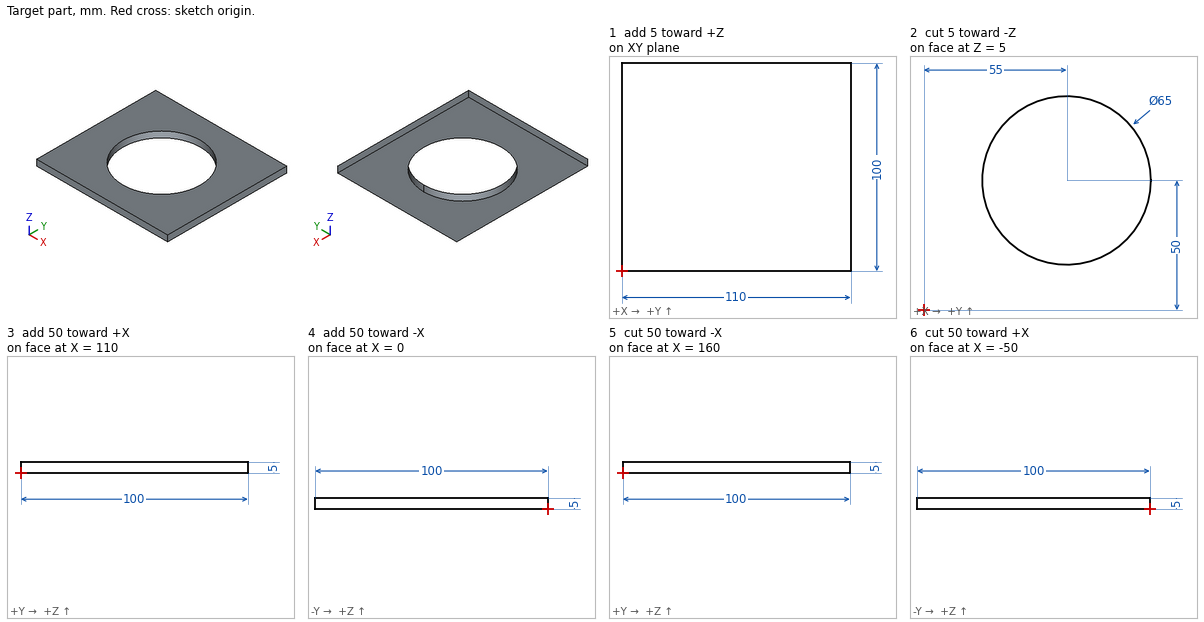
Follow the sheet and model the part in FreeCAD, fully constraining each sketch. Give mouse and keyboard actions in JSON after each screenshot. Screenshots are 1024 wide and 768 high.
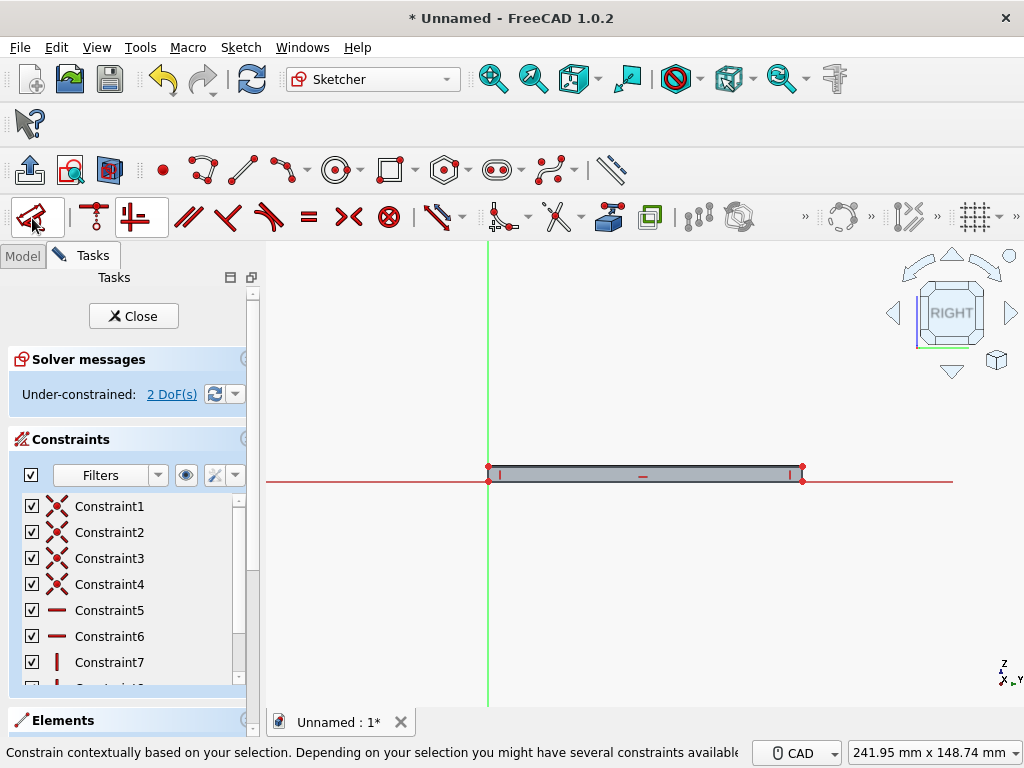
{"action": "scroll", "coordinate": [802, 474], "scroll_direction": "up", "scroll_amount": 5}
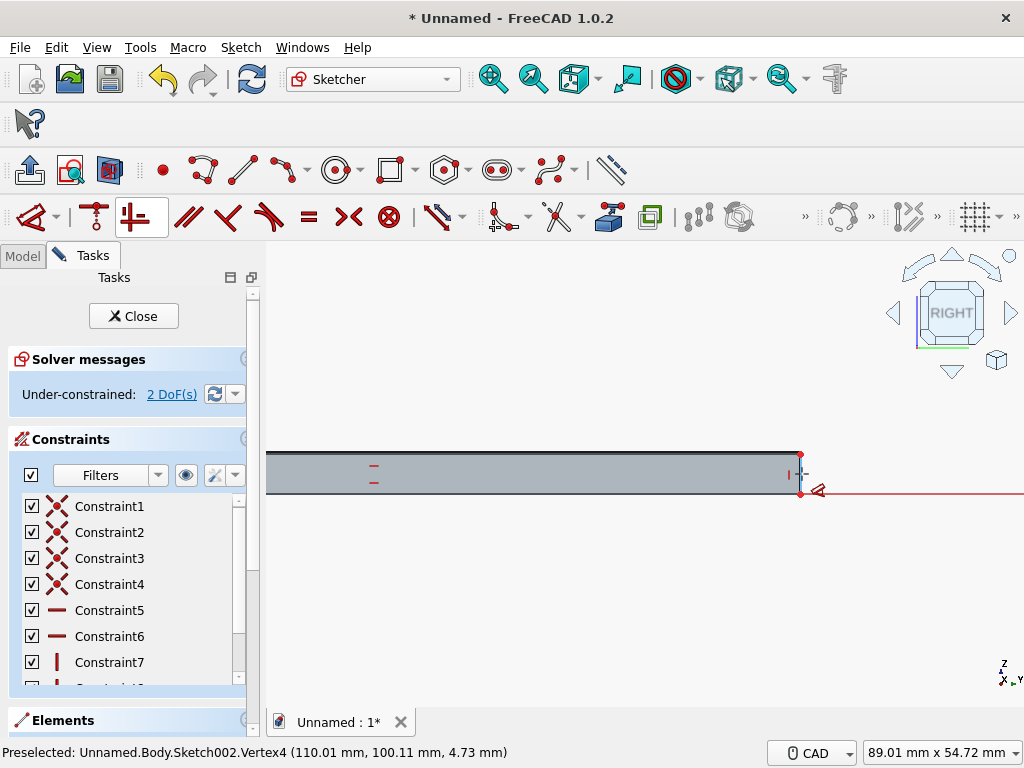
{"action": "left_click", "coordinate": [801, 474]}
{"action": "left_click", "coordinate": [835, 474]}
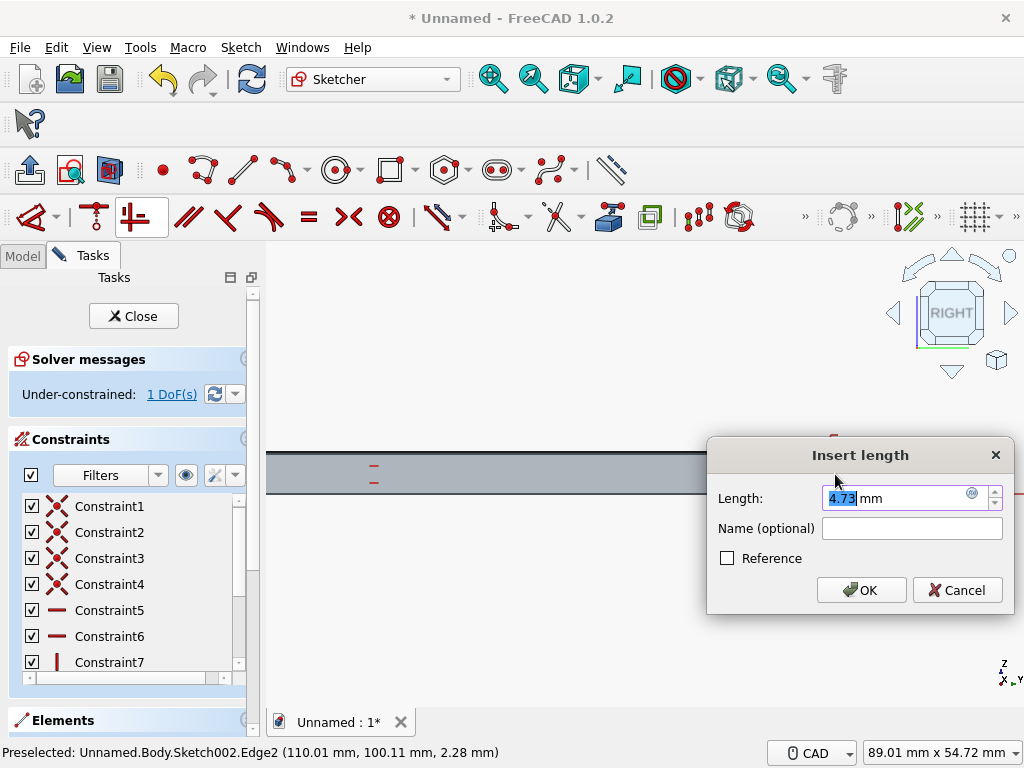
{"action": "type", "text": "5"}
{"action": "key", "text": "Return"}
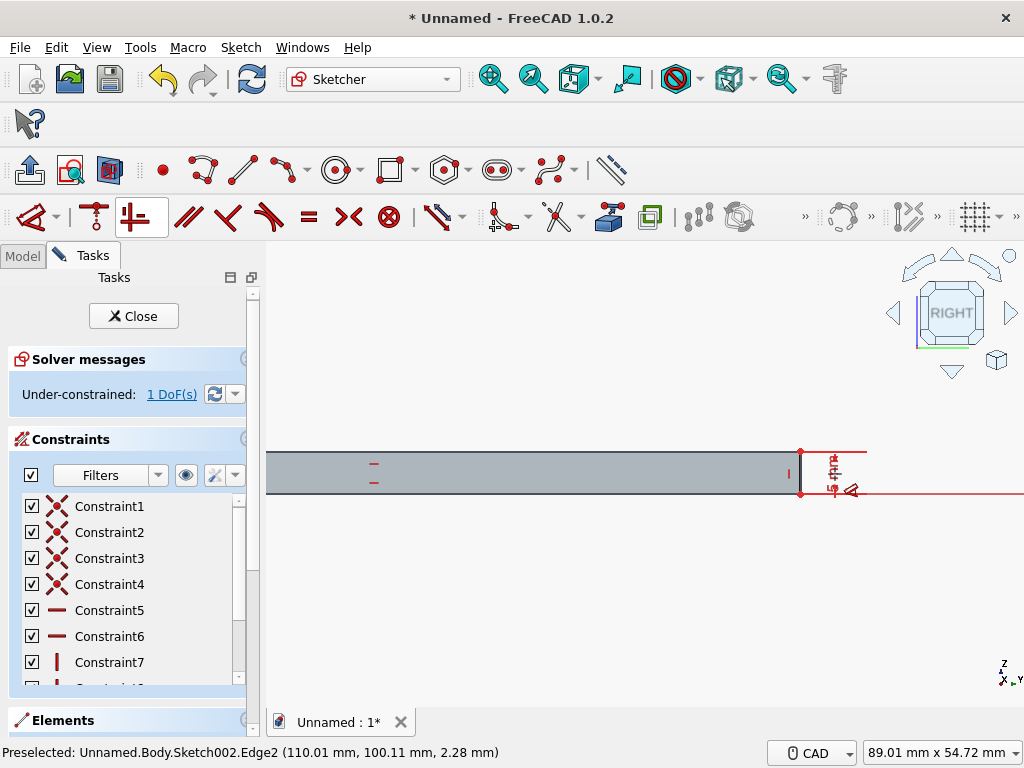
{"action": "left_click", "coordinate": [545, 494]}
{"action": "left_click", "coordinate": [547, 528]}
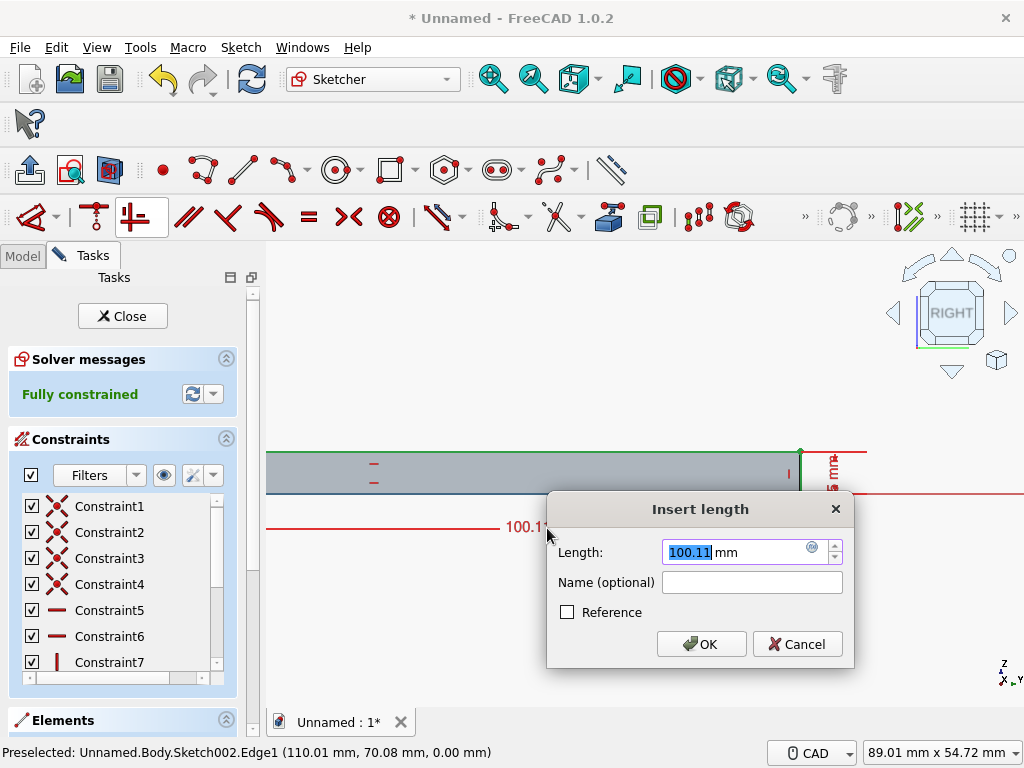
{"action": "type", "text": "100"}
{"action": "key", "text": "Return"}
{"action": "key", "text": "Escape"}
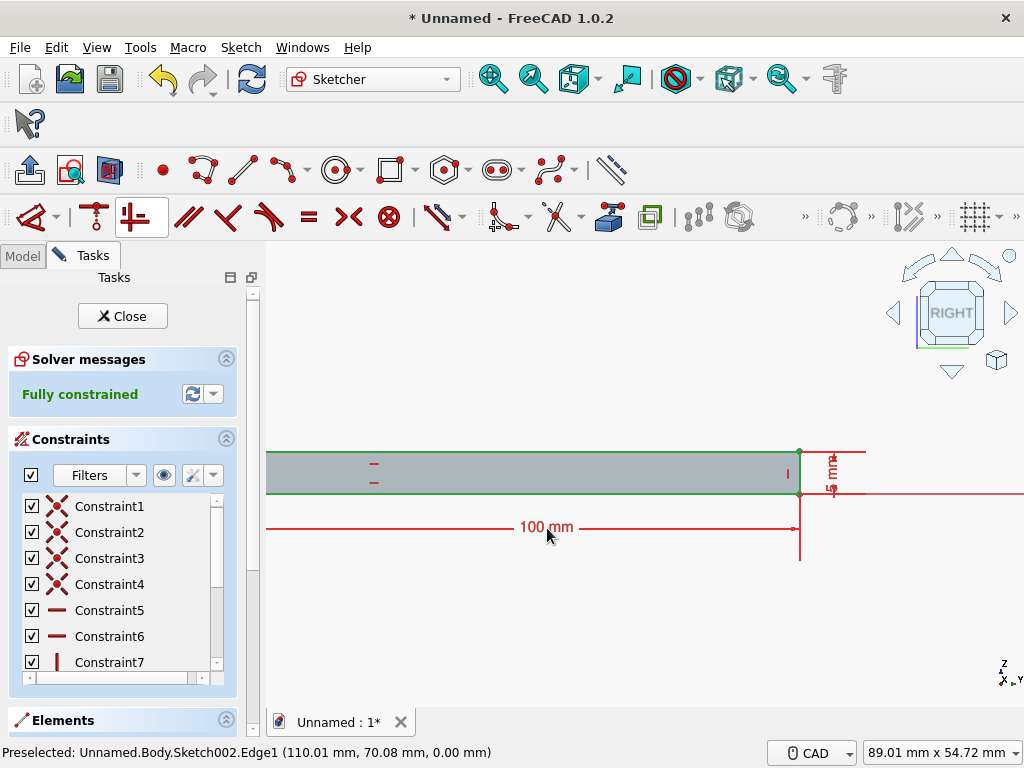
{"action": "left_click", "coordinate": [123, 316]}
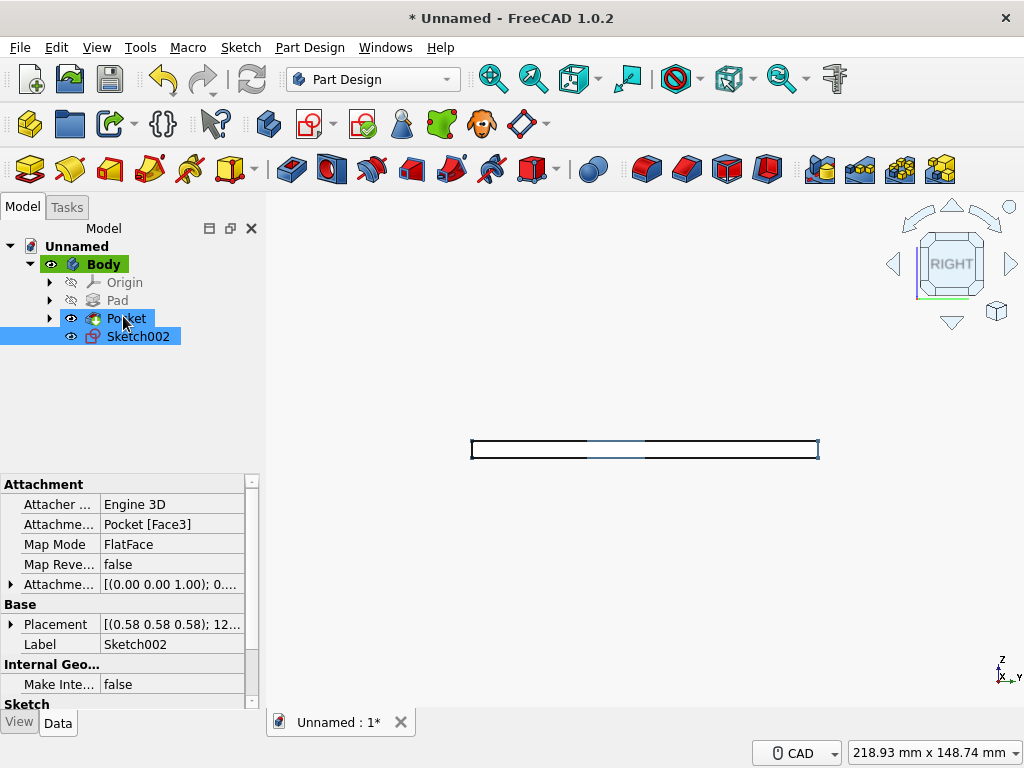
{"action": "left_click", "coordinate": [30, 170]}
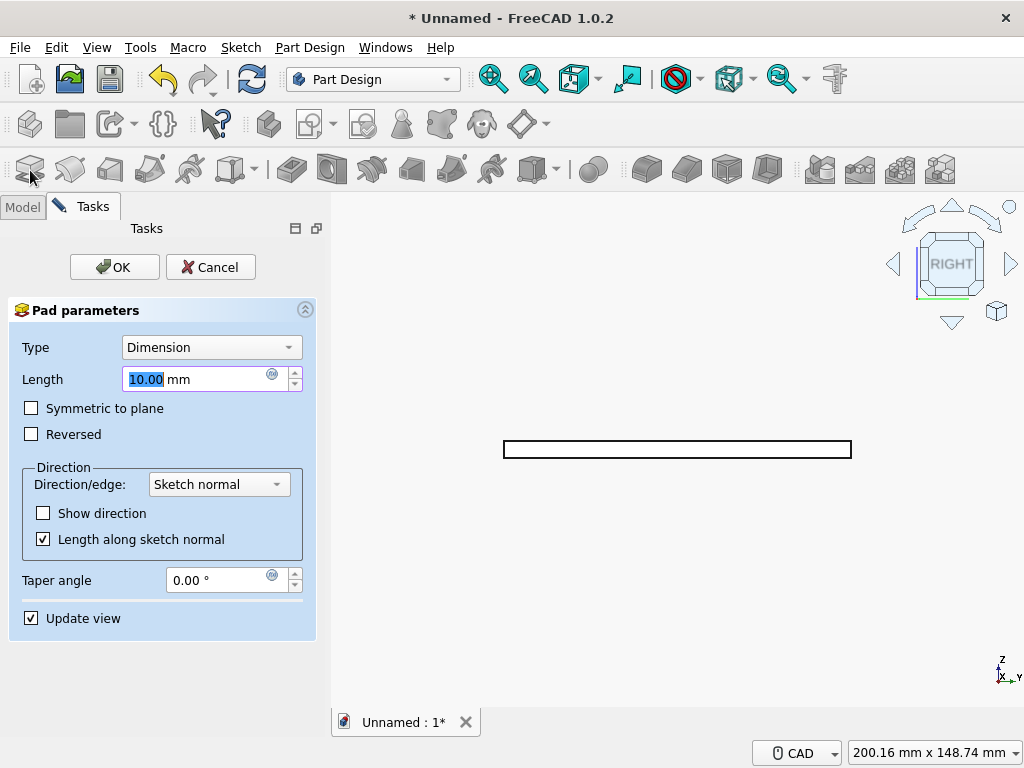
{"action": "type", "text": "50"}
{"action": "key", "text": "Tab"}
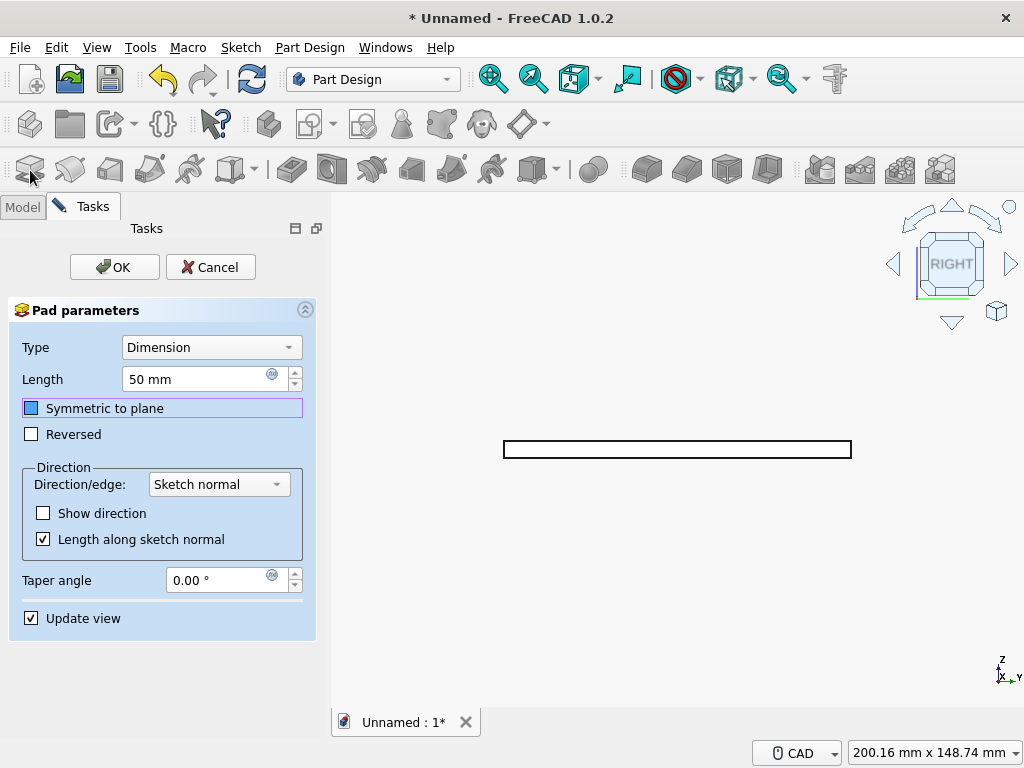
{"action": "left_click", "coordinate": [115, 267]}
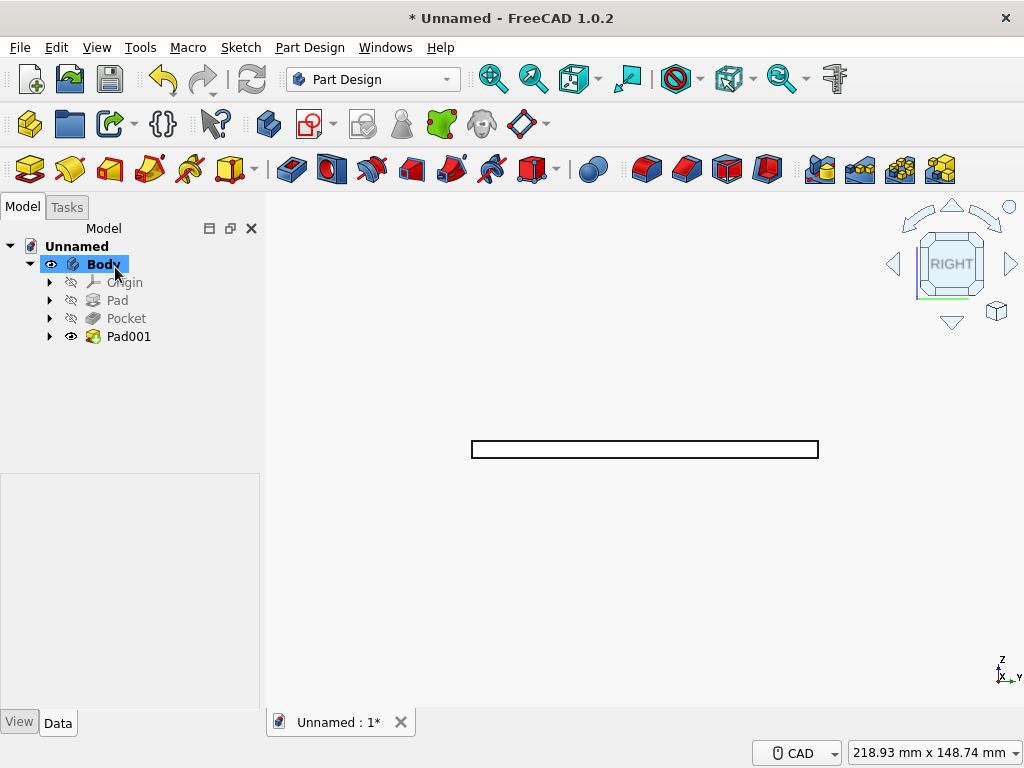
{"action": "key", "text": "6"}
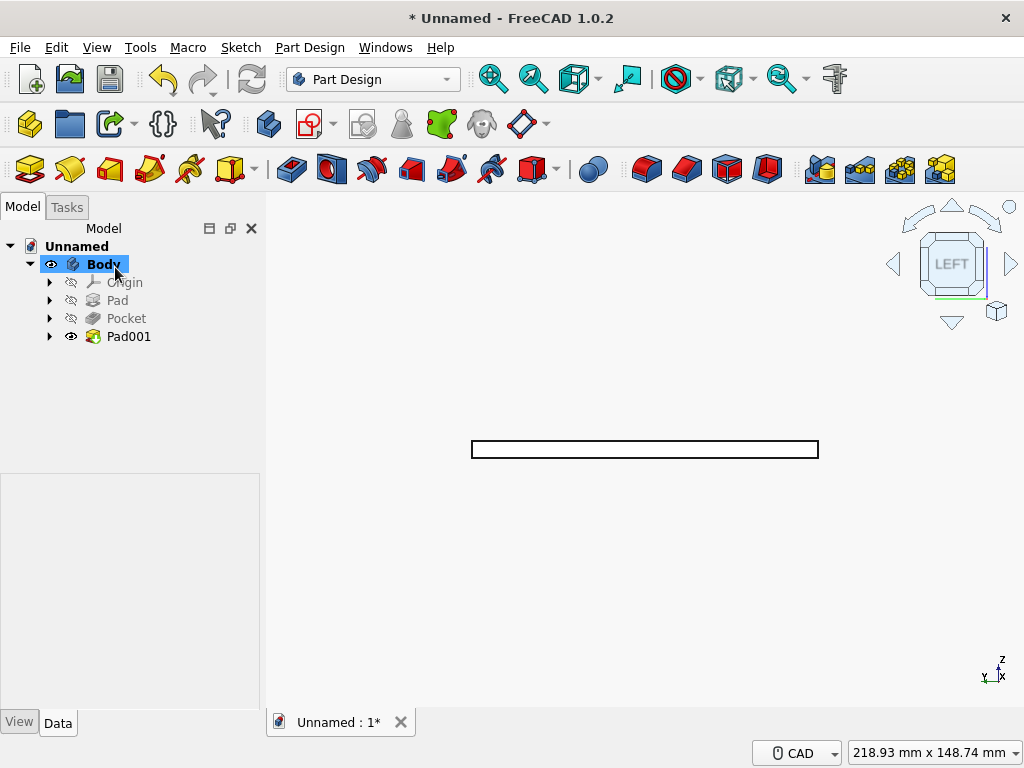
{"action": "left_click", "coordinate": [497, 449]}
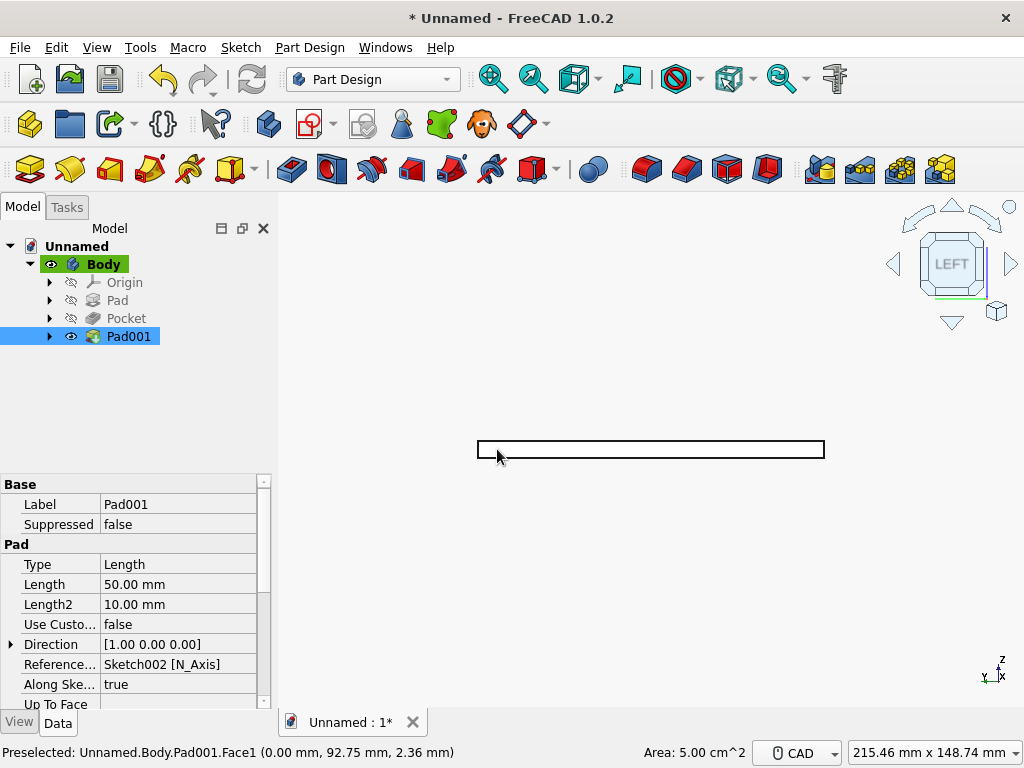
{"action": "left_click", "coordinate": [310, 124]}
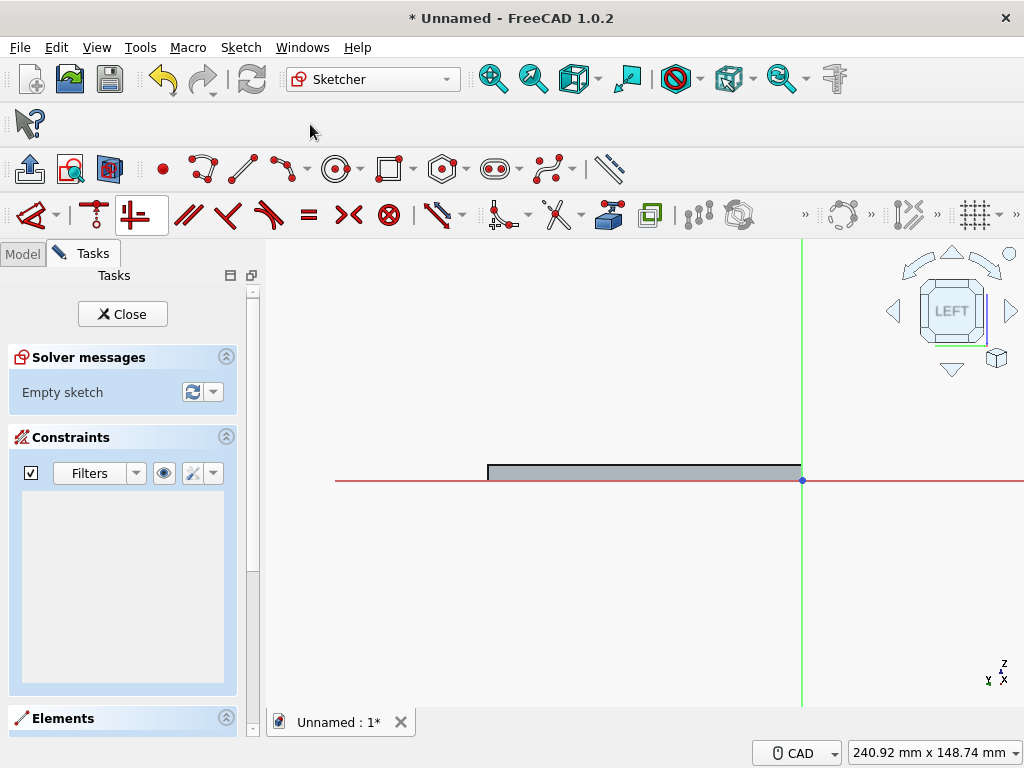
{"action": "left_click", "coordinate": [390, 170]}